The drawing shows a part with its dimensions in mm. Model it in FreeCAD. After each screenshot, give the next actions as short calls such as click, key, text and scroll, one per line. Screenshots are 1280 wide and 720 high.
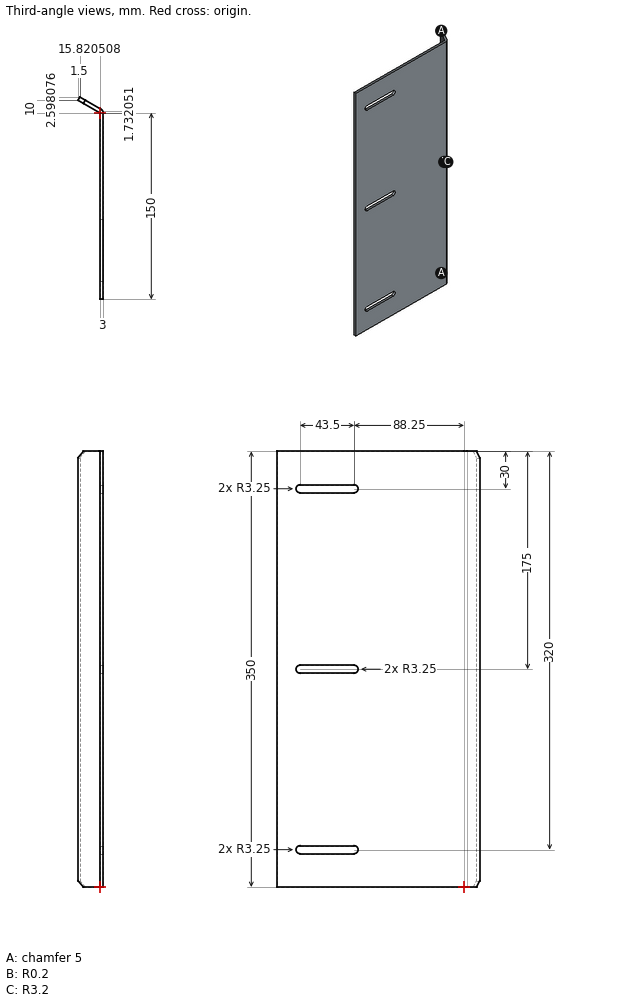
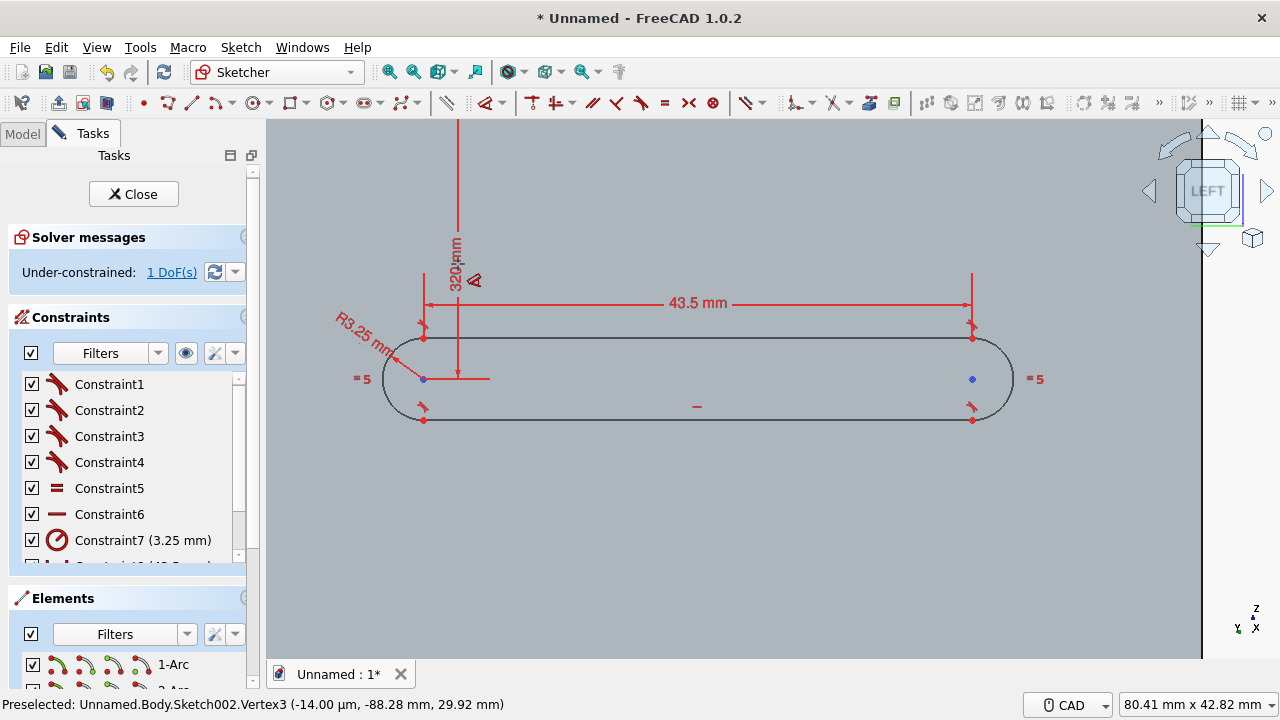
click(424, 338)
click(359, 372)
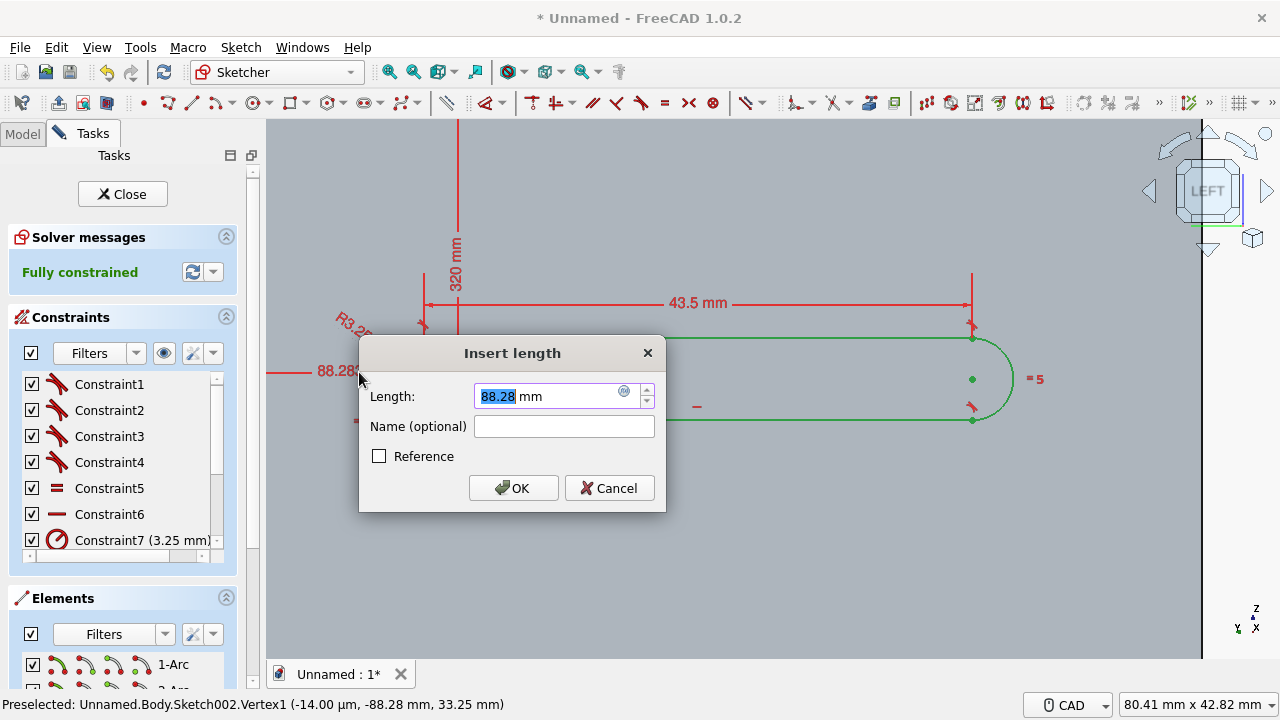
text(88.25)
key(Return)
key(Escape)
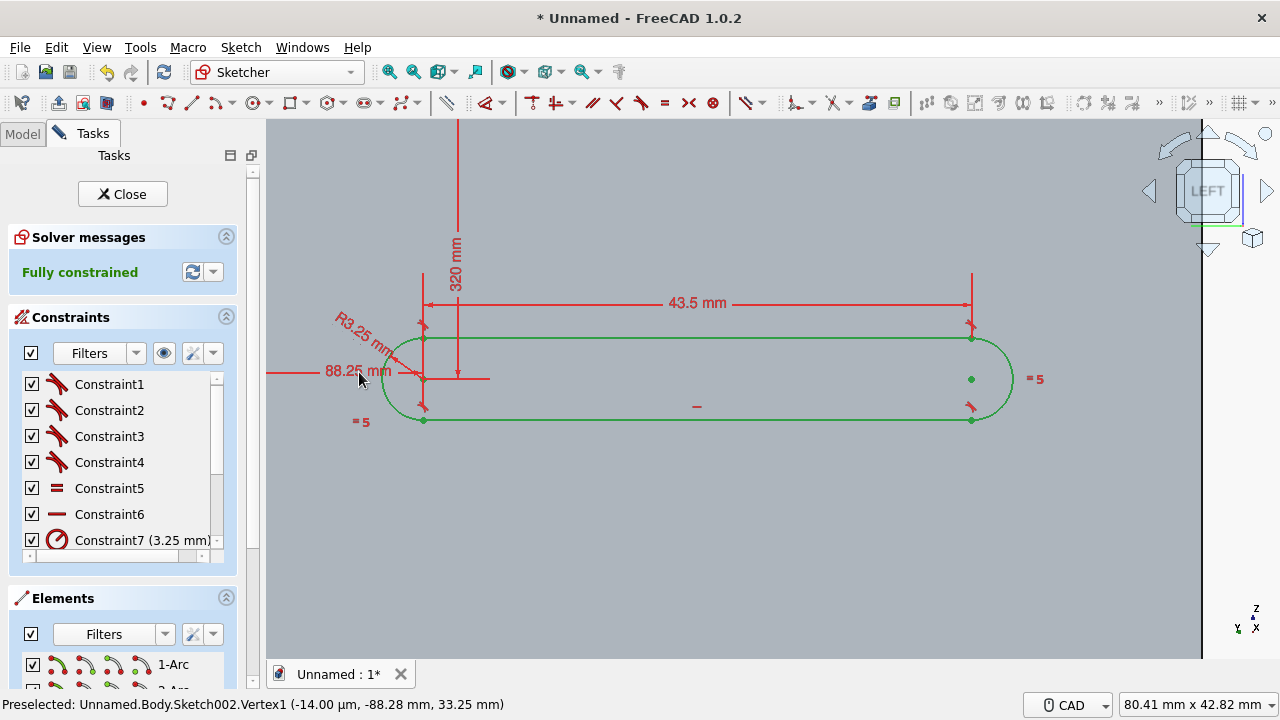
click(123, 194)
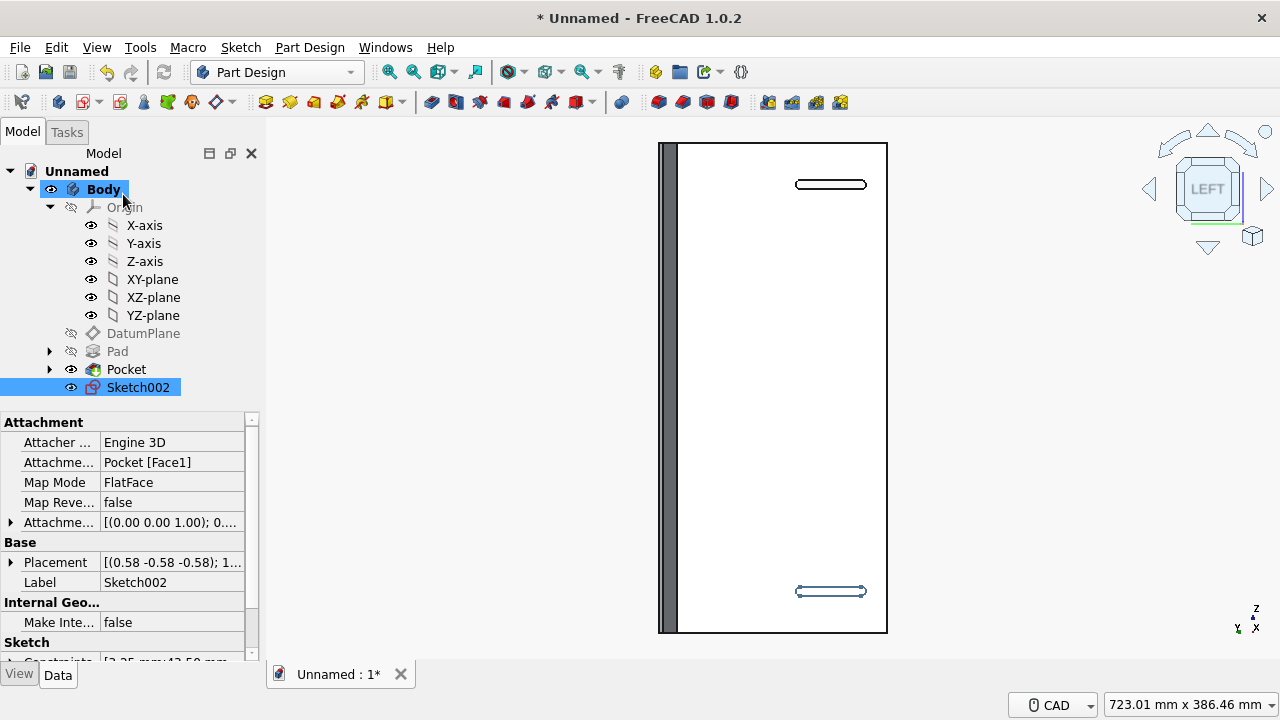
click(432, 102)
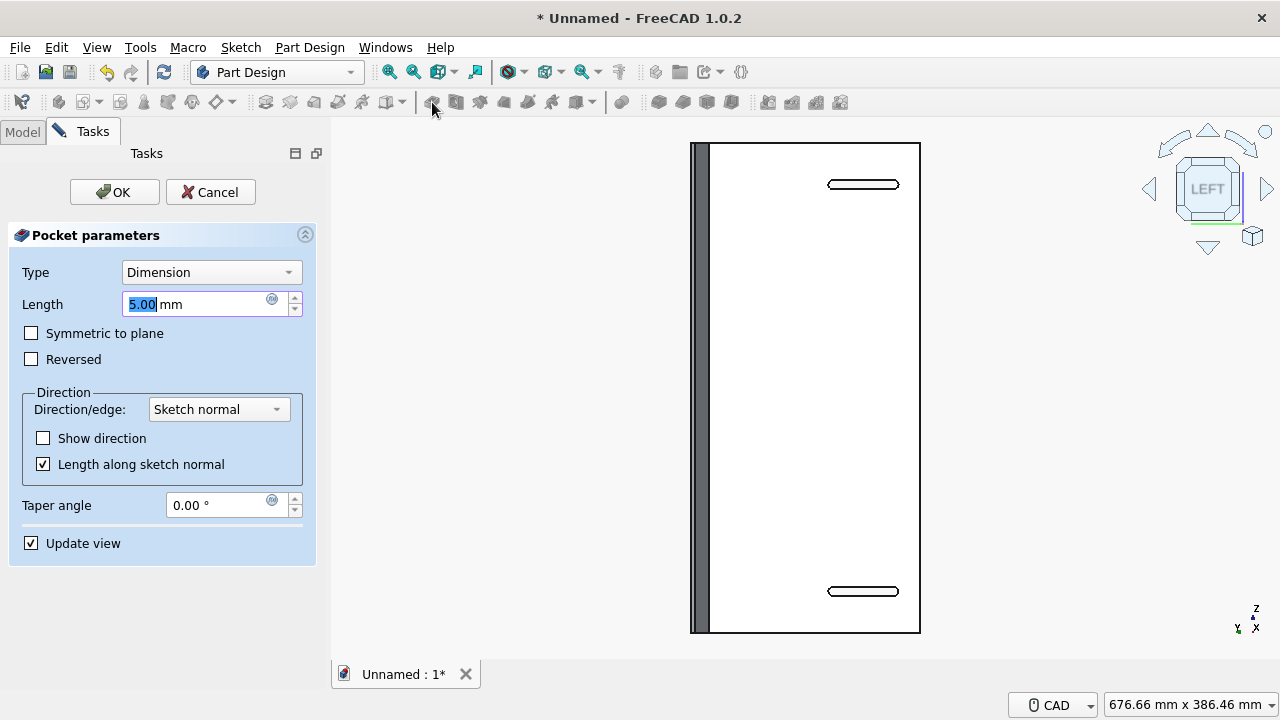
click(212, 272)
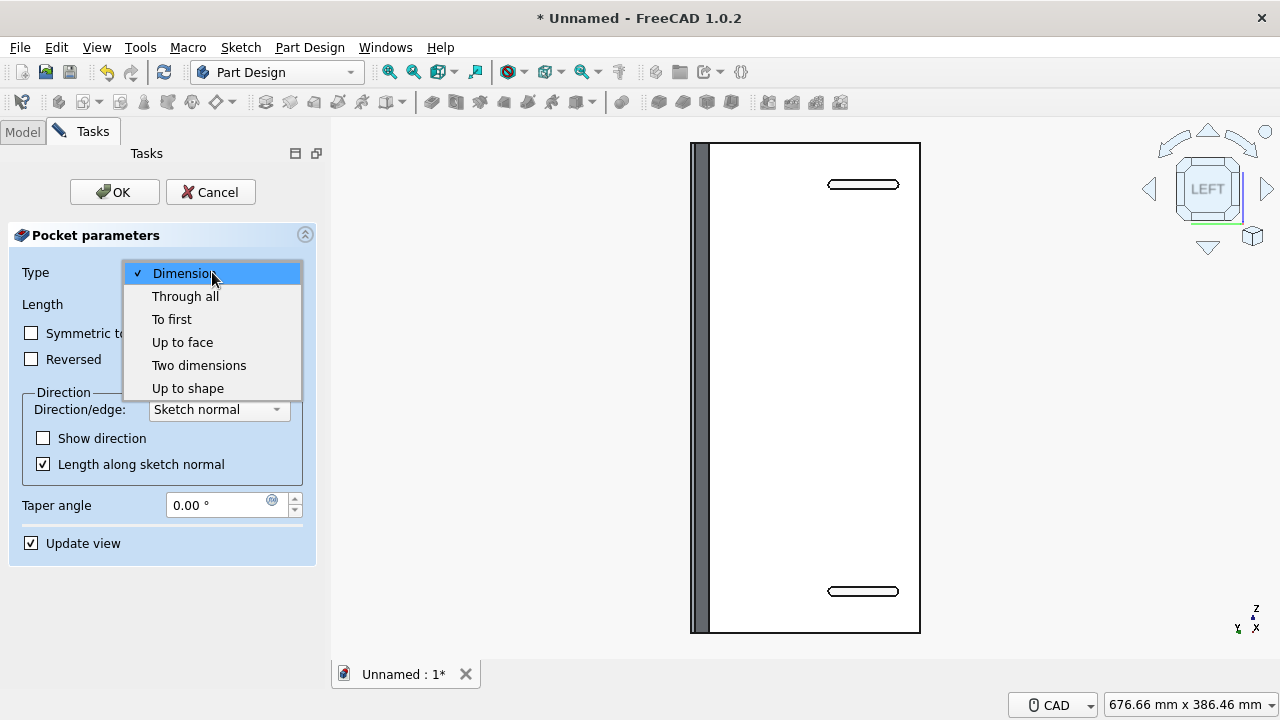
click(212, 296)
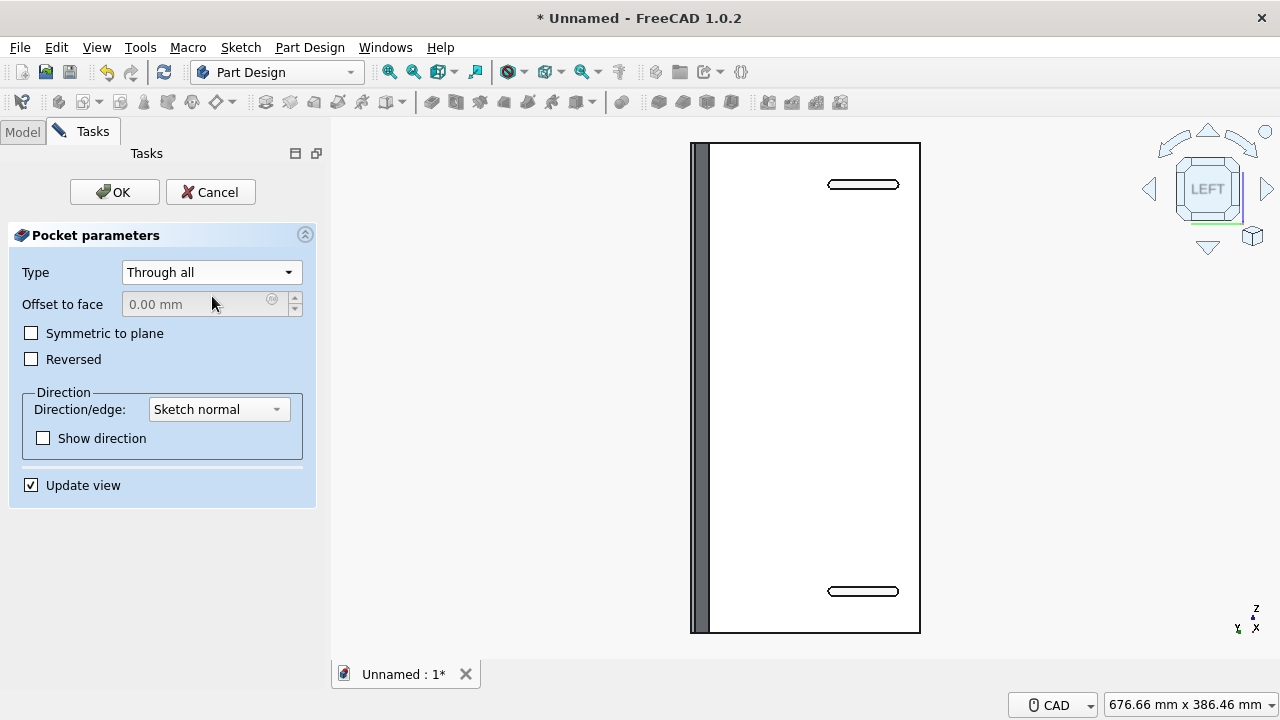
click(115, 192)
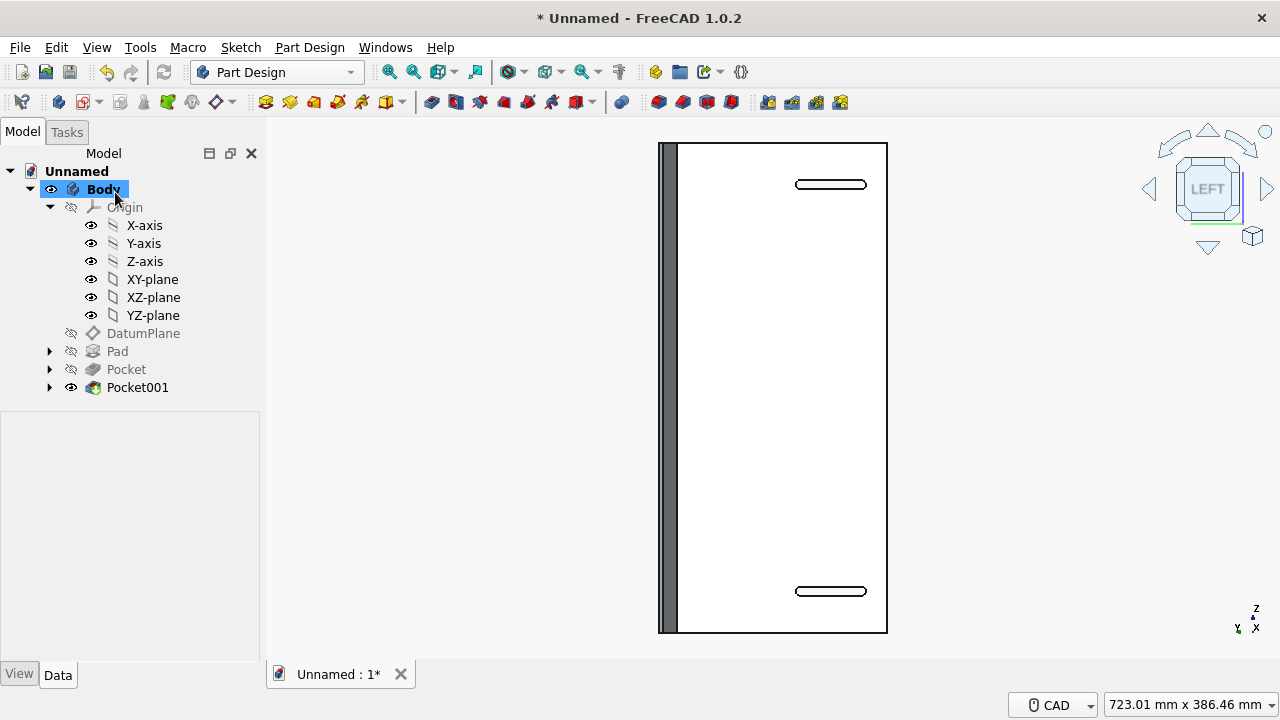
key(0)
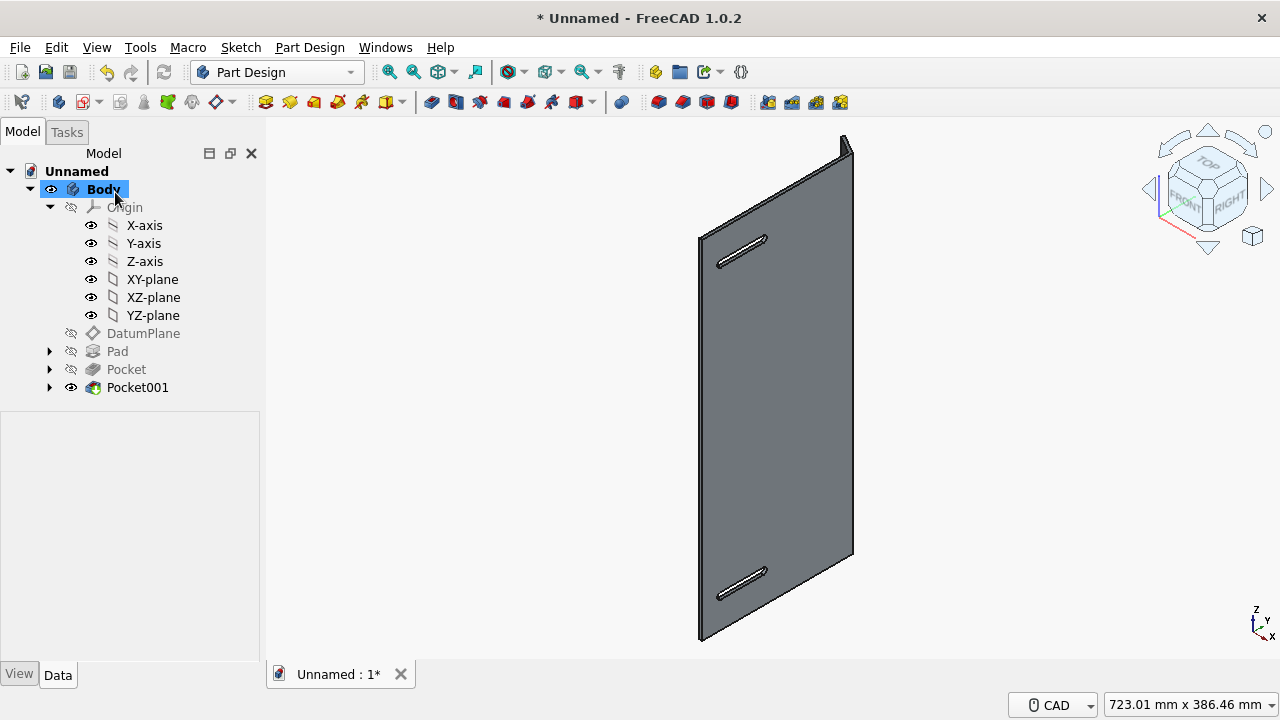
click(778, 339)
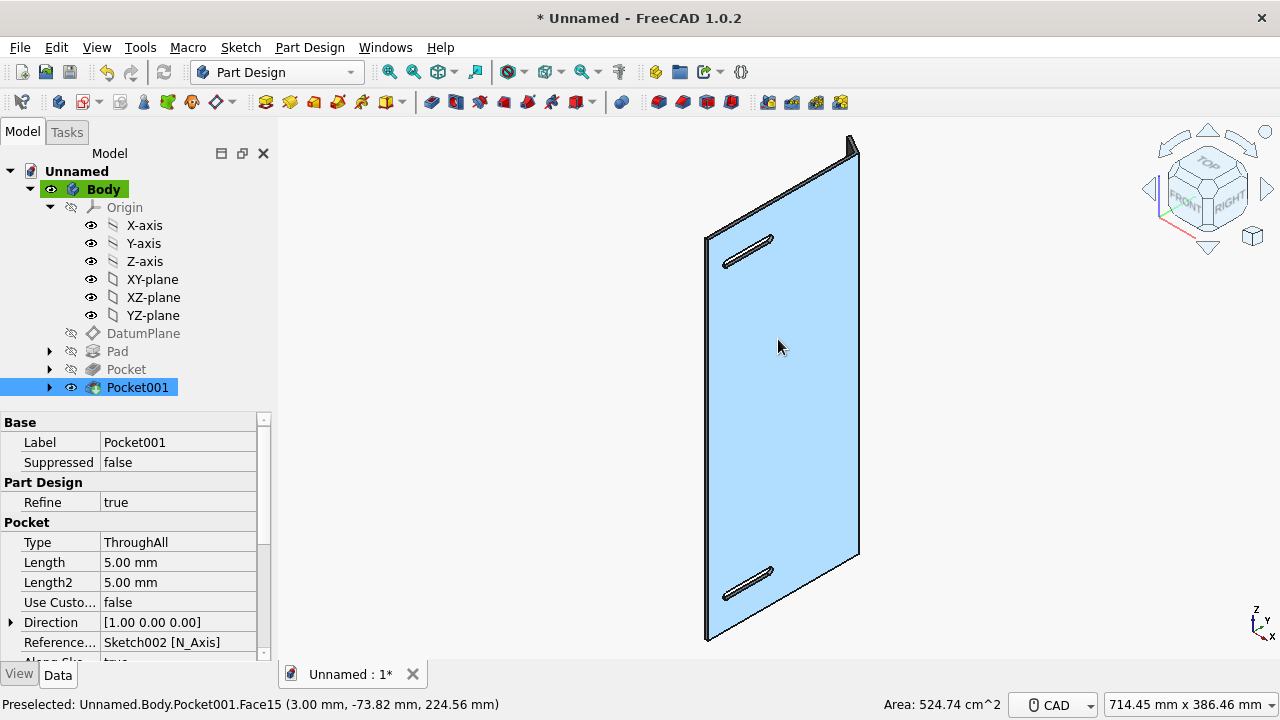
click(84, 102)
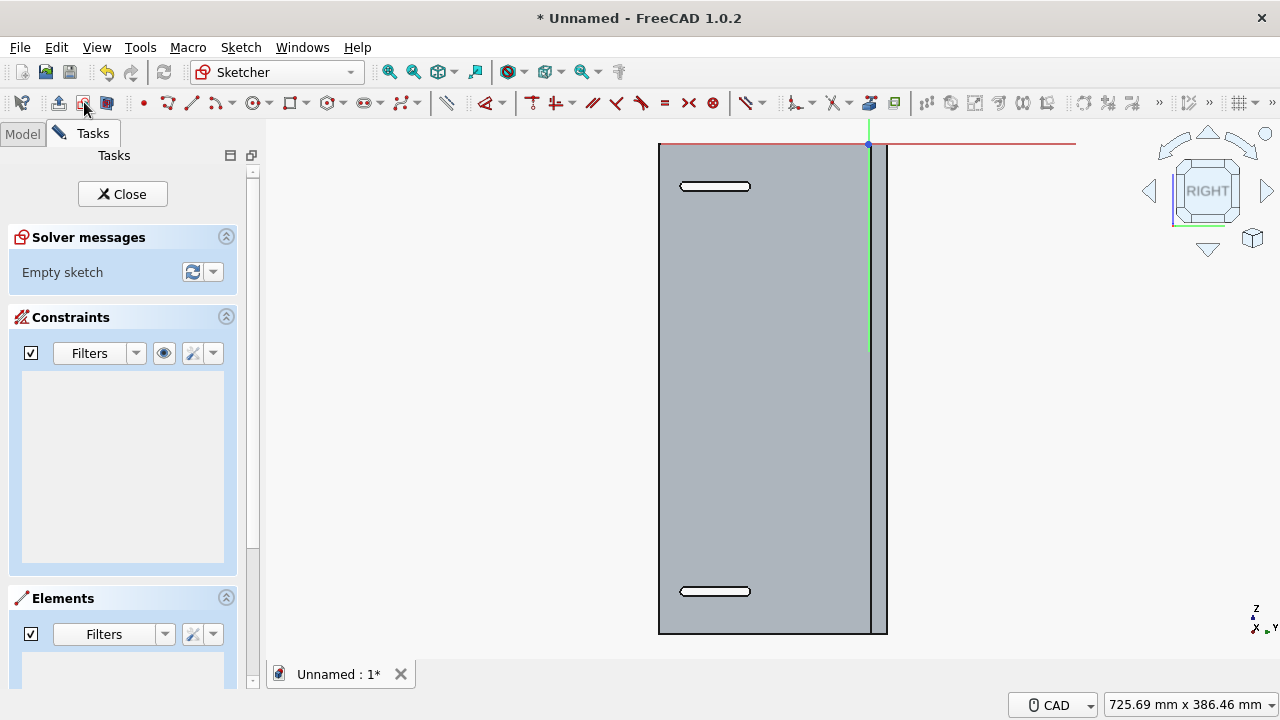
scroll(717, 389, up, 11)